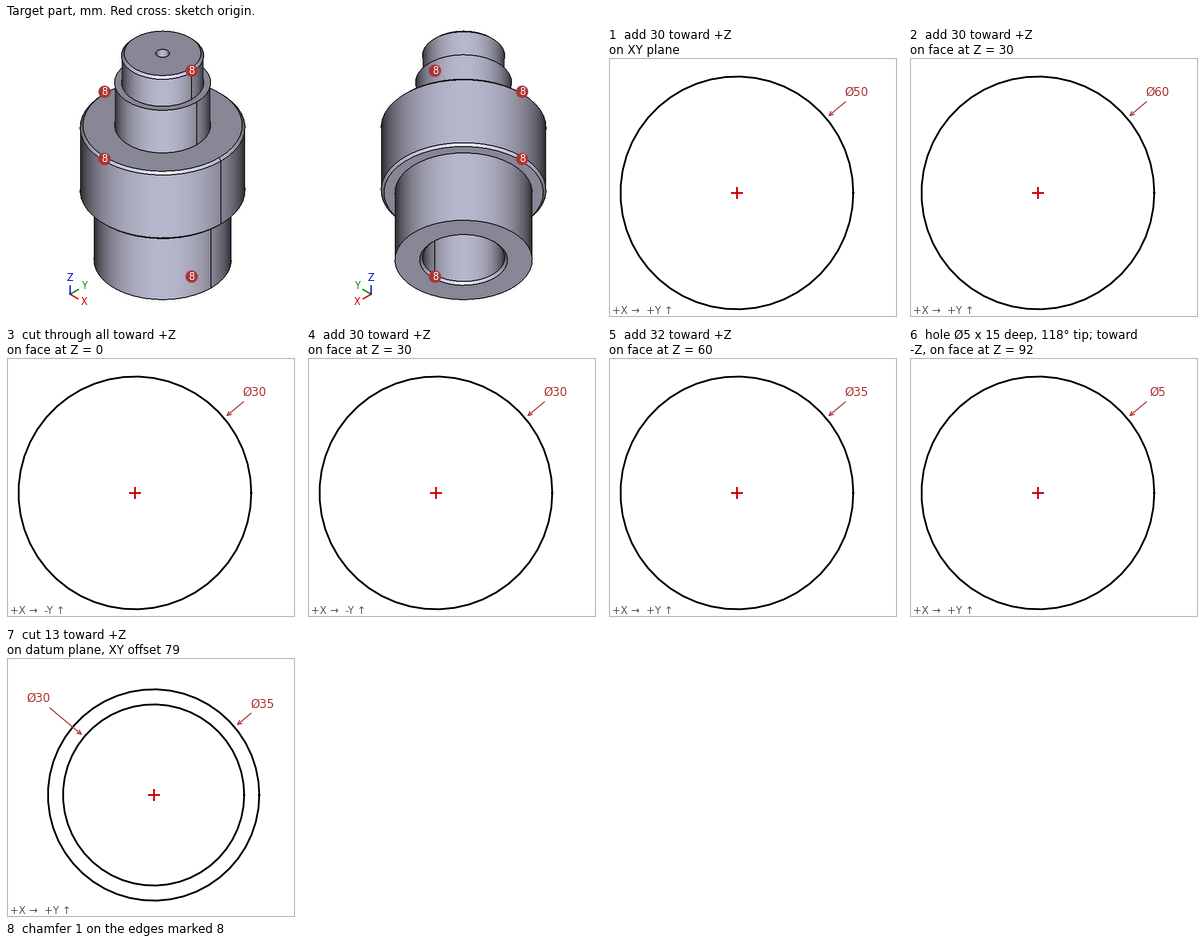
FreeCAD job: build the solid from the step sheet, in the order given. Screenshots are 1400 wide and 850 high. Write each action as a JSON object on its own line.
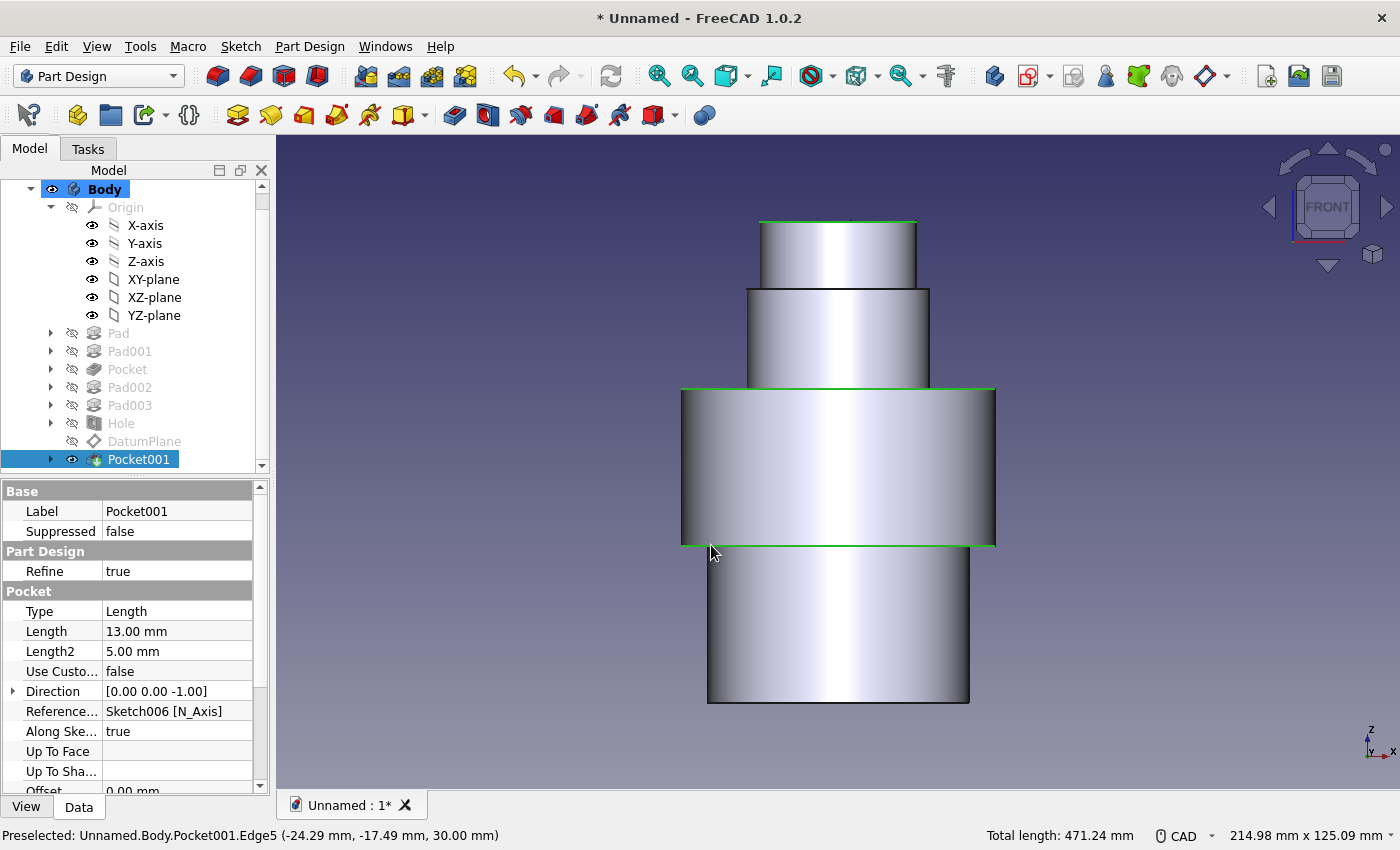
{"action": "key", "text": "3"}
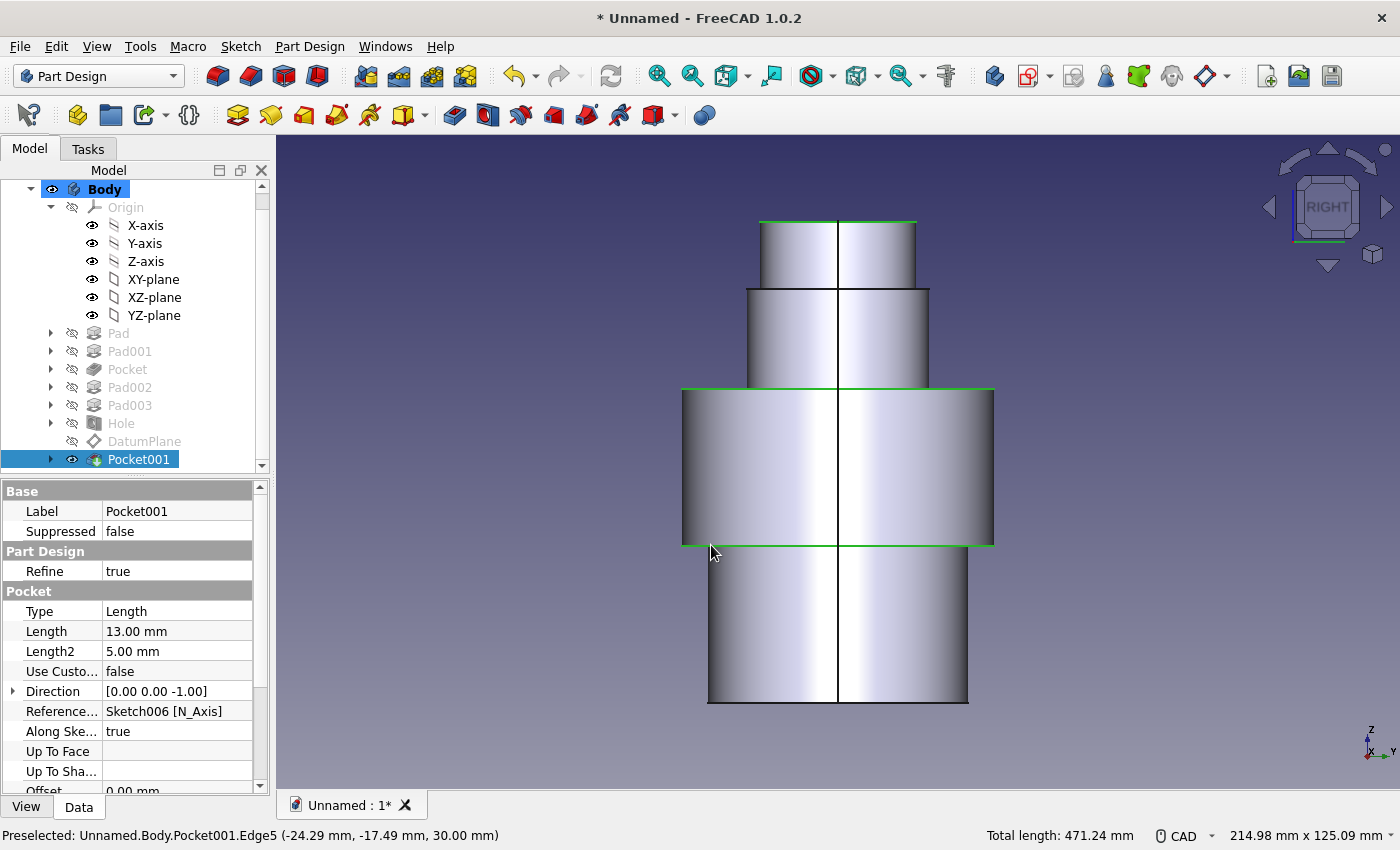
{"action": "key", "text": "5"}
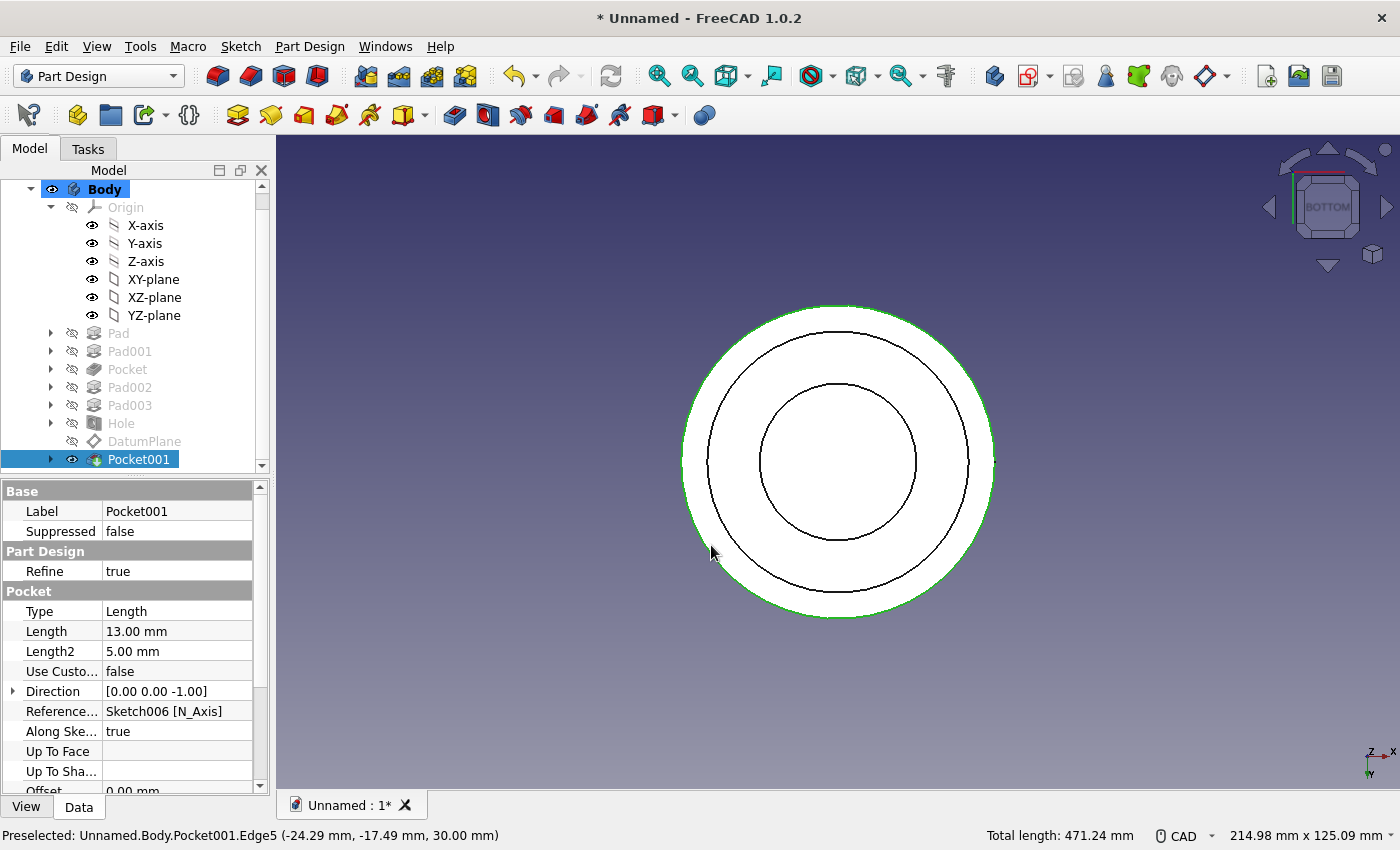
{"action": "left_click", "coordinate": [760, 461], "text": "ctrl"}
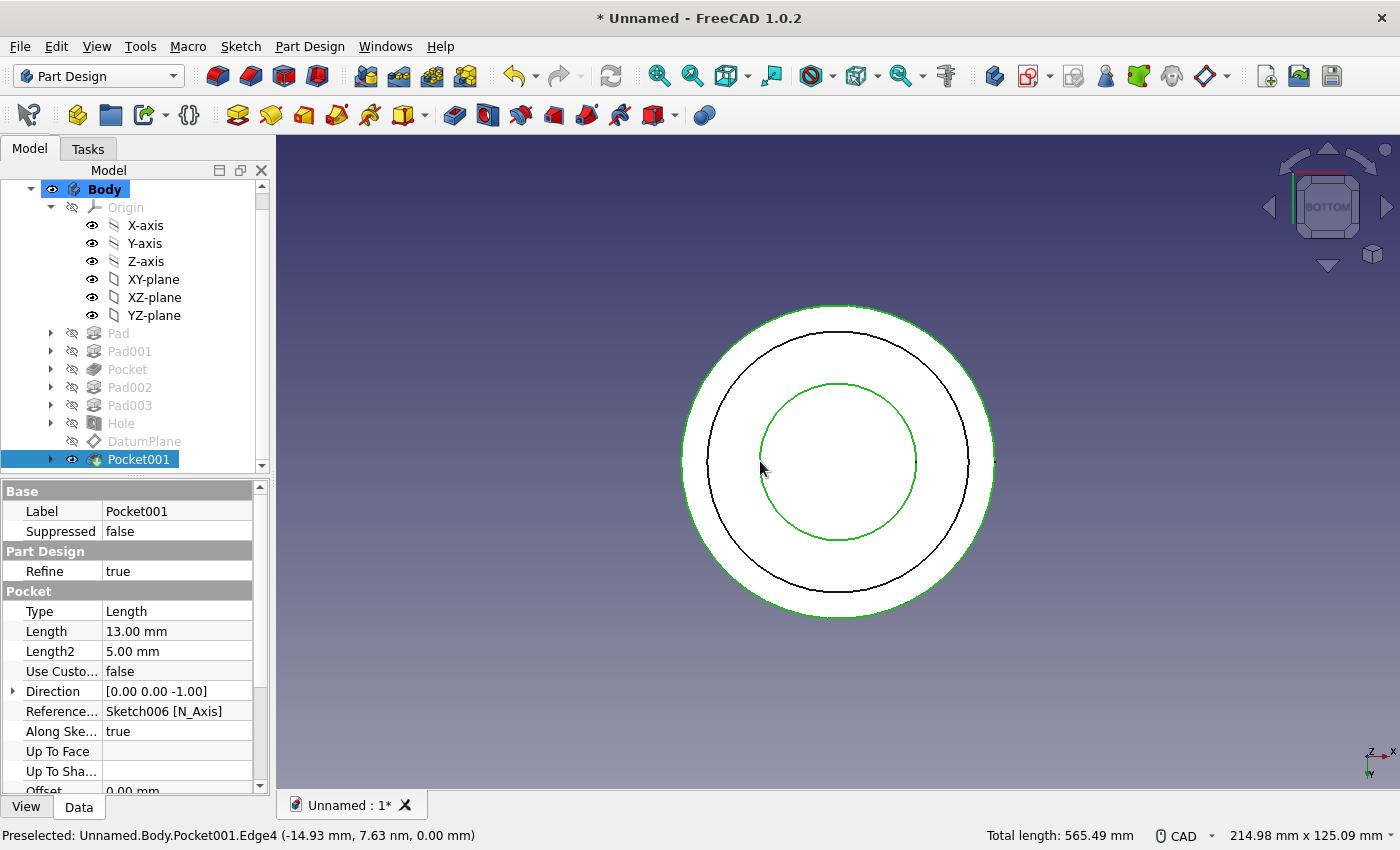
{"action": "left_click", "coordinate": [251, 76]}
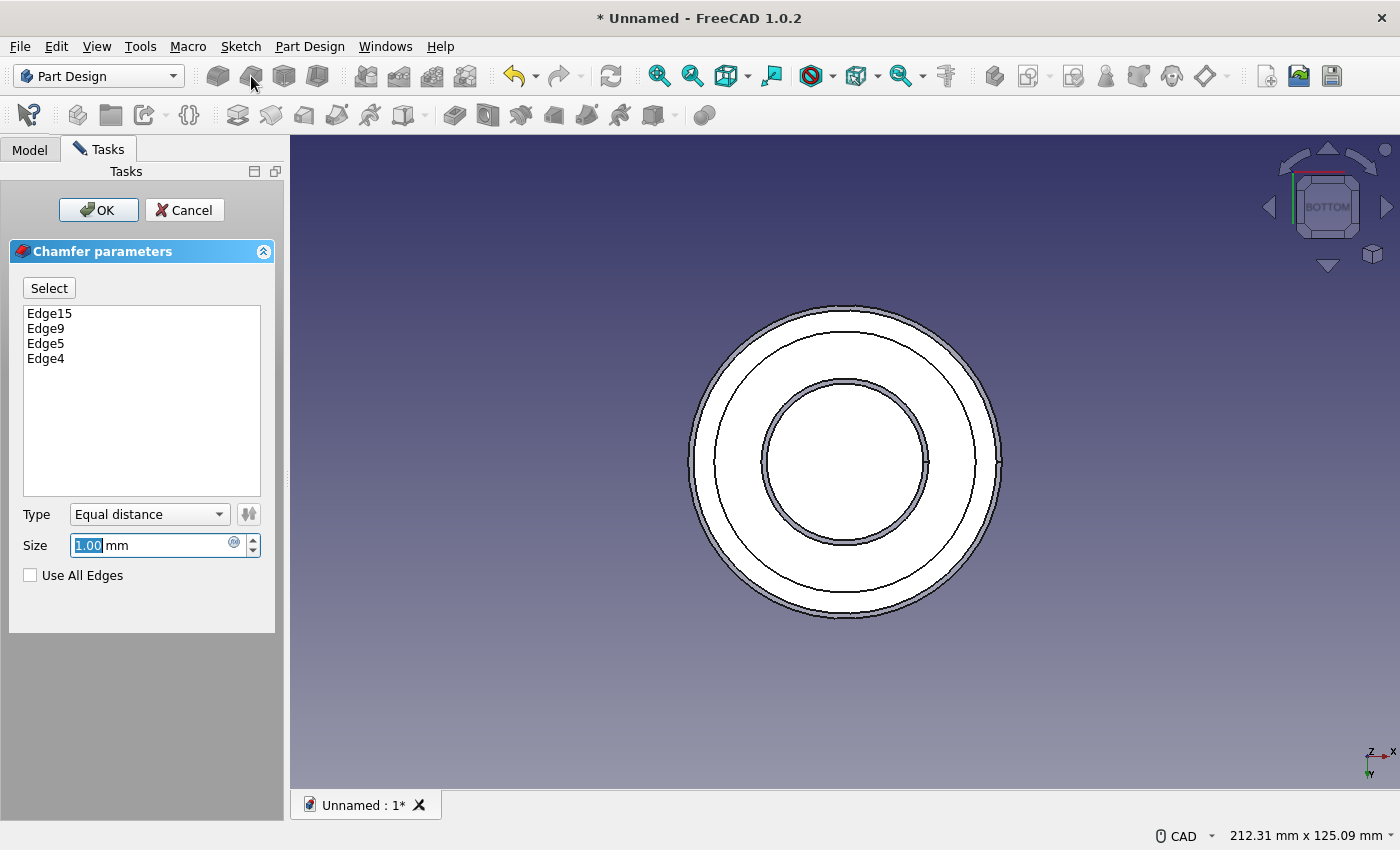
{"action": "type", "text": "1"}
{"action": "key", "text": "Tab"}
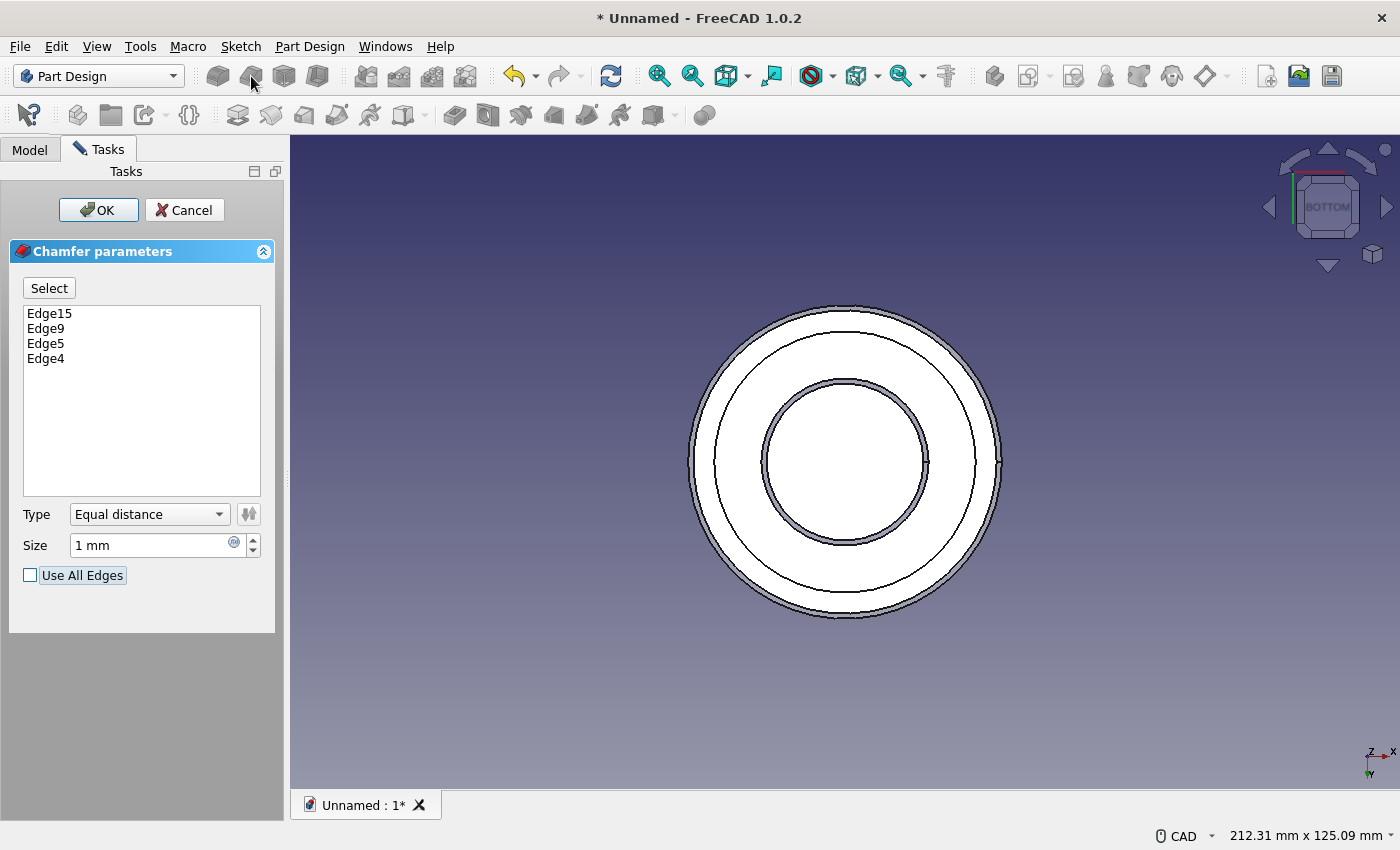
{"action": "left_click", "coordinate": [99, 210]}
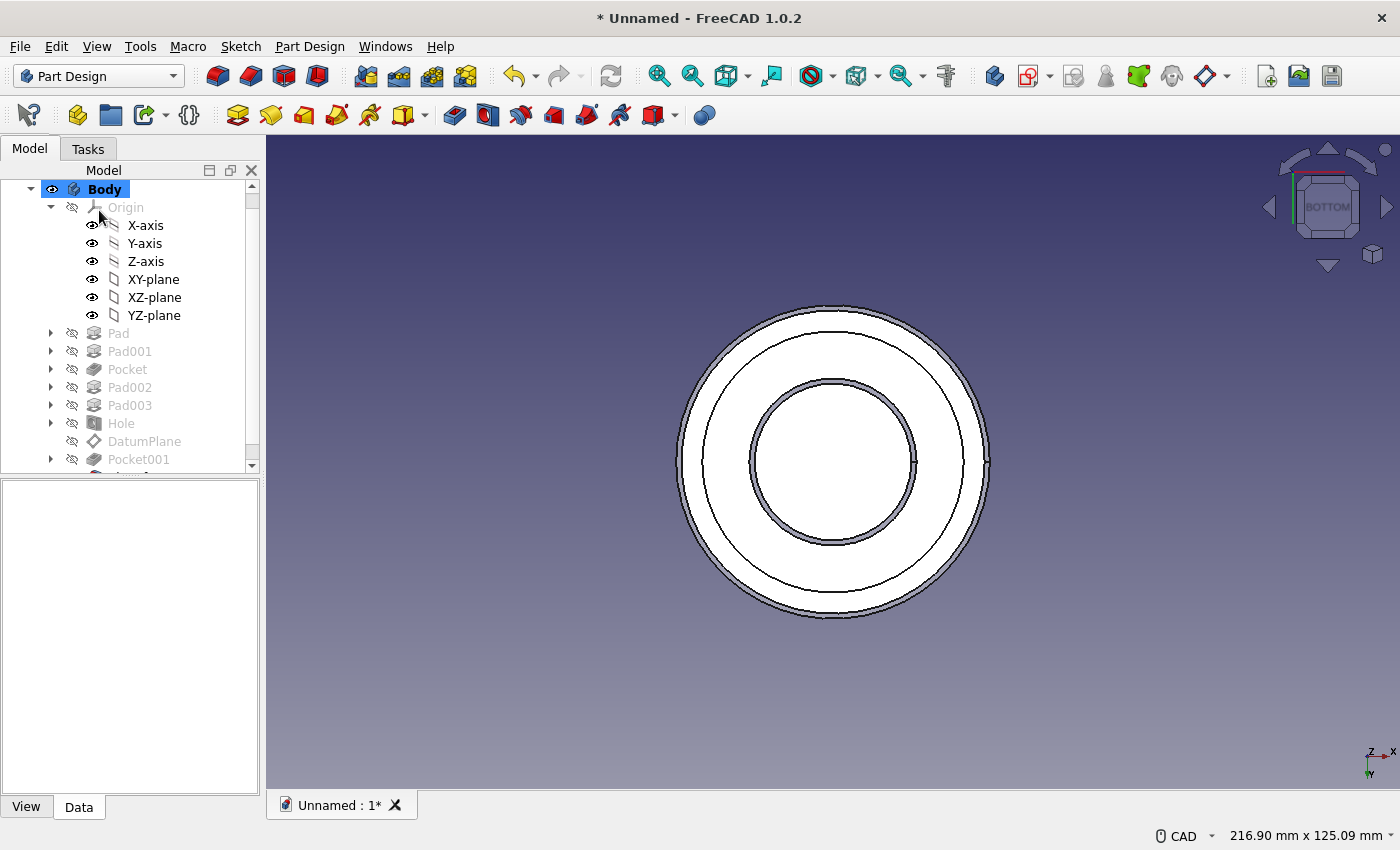
{"action": "key", "text": "0"}